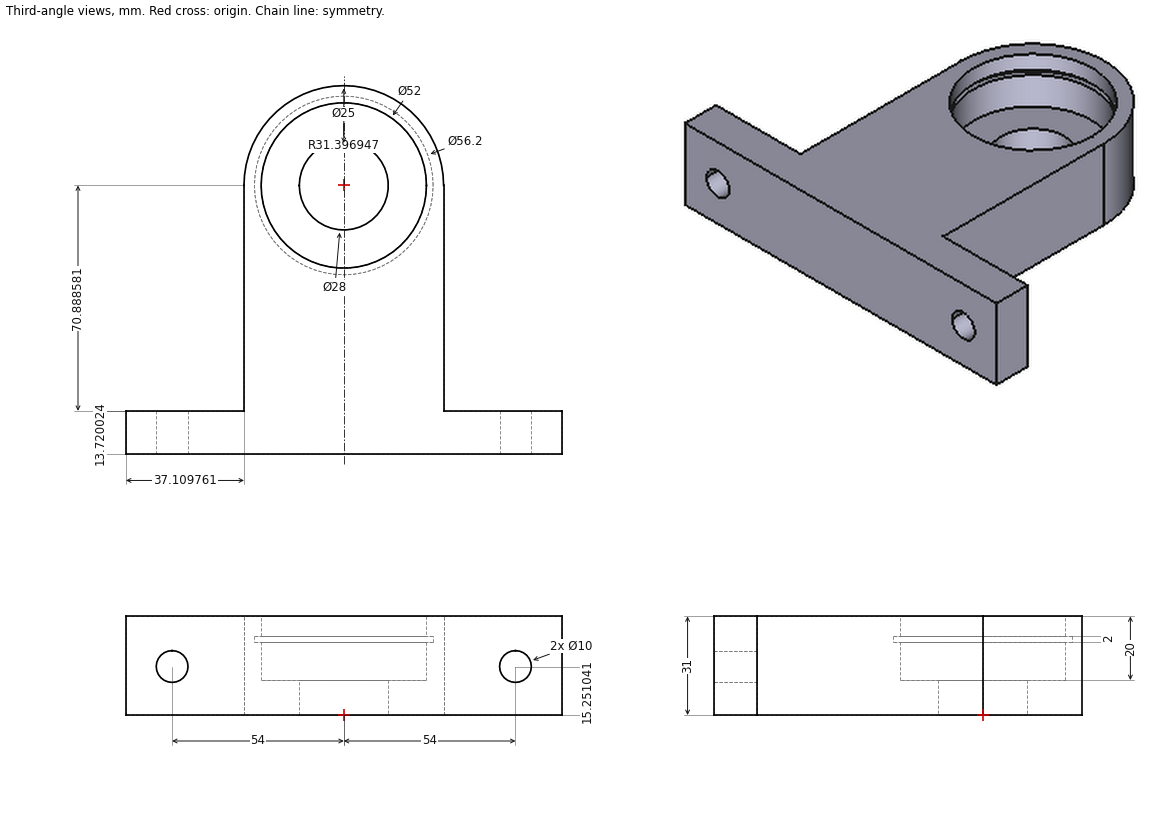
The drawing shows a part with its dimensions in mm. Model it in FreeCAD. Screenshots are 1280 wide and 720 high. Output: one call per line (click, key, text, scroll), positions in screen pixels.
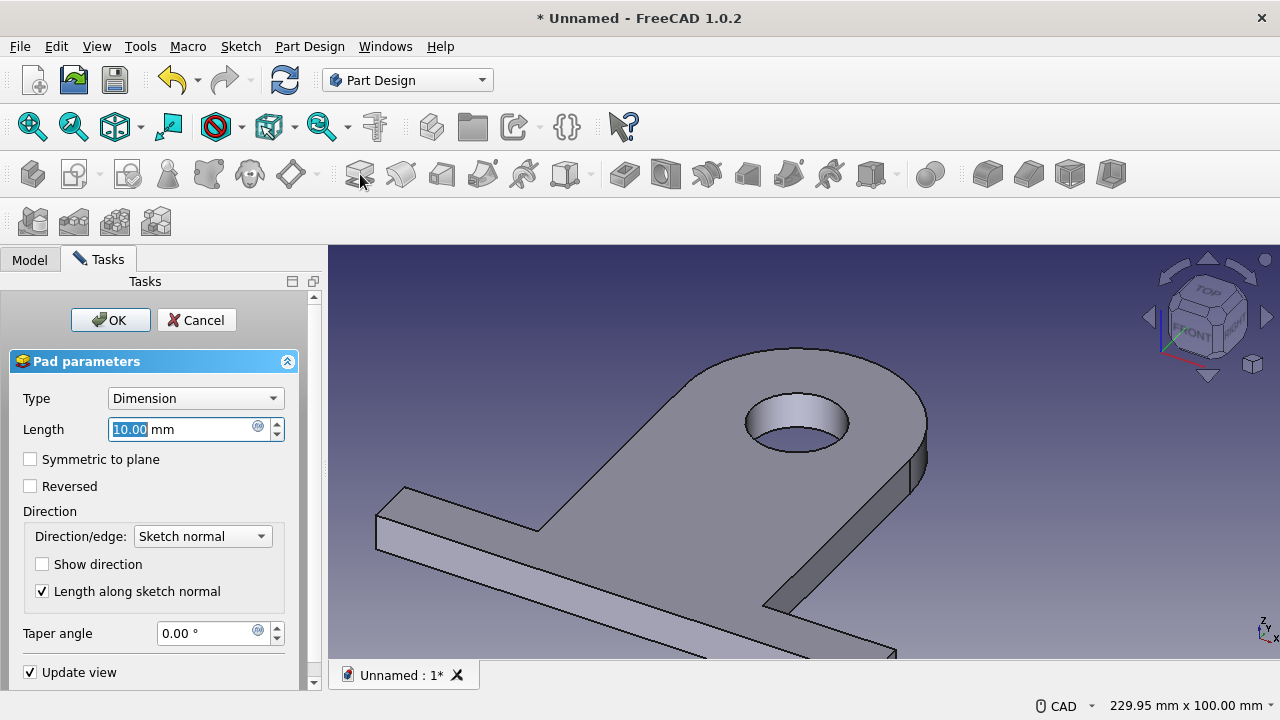
text(31)
key(Tab)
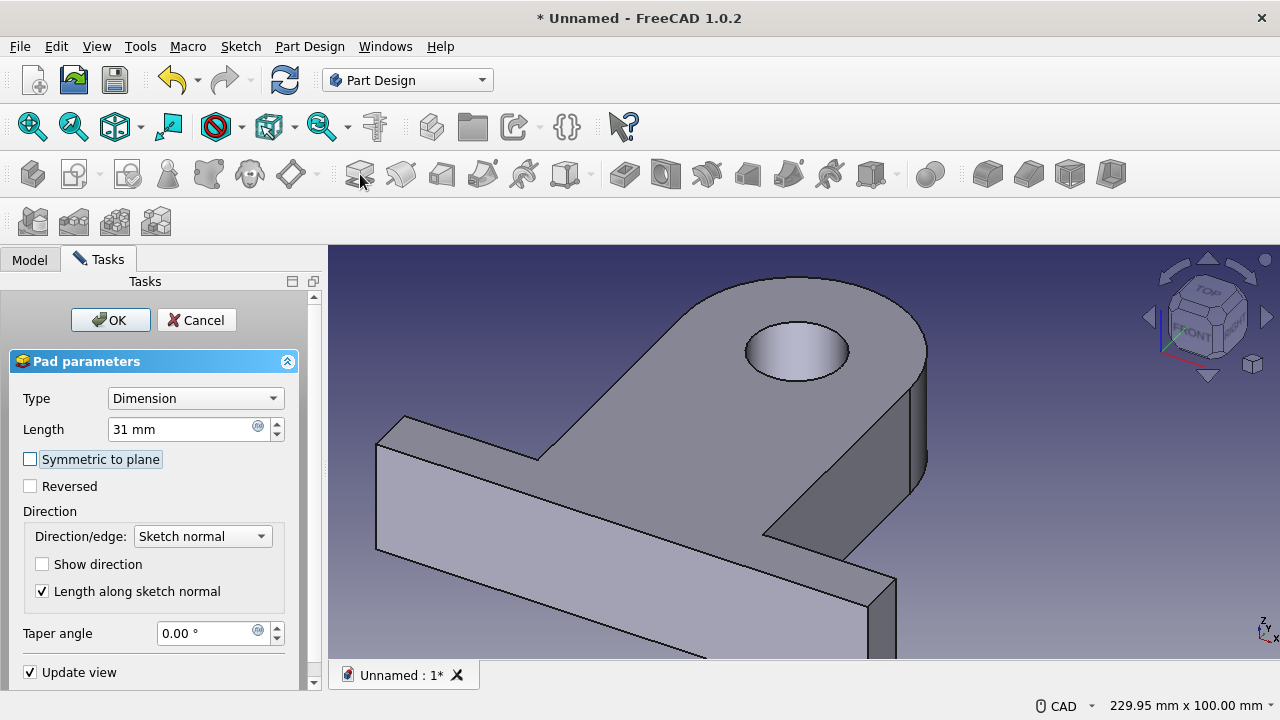
click(111, 320)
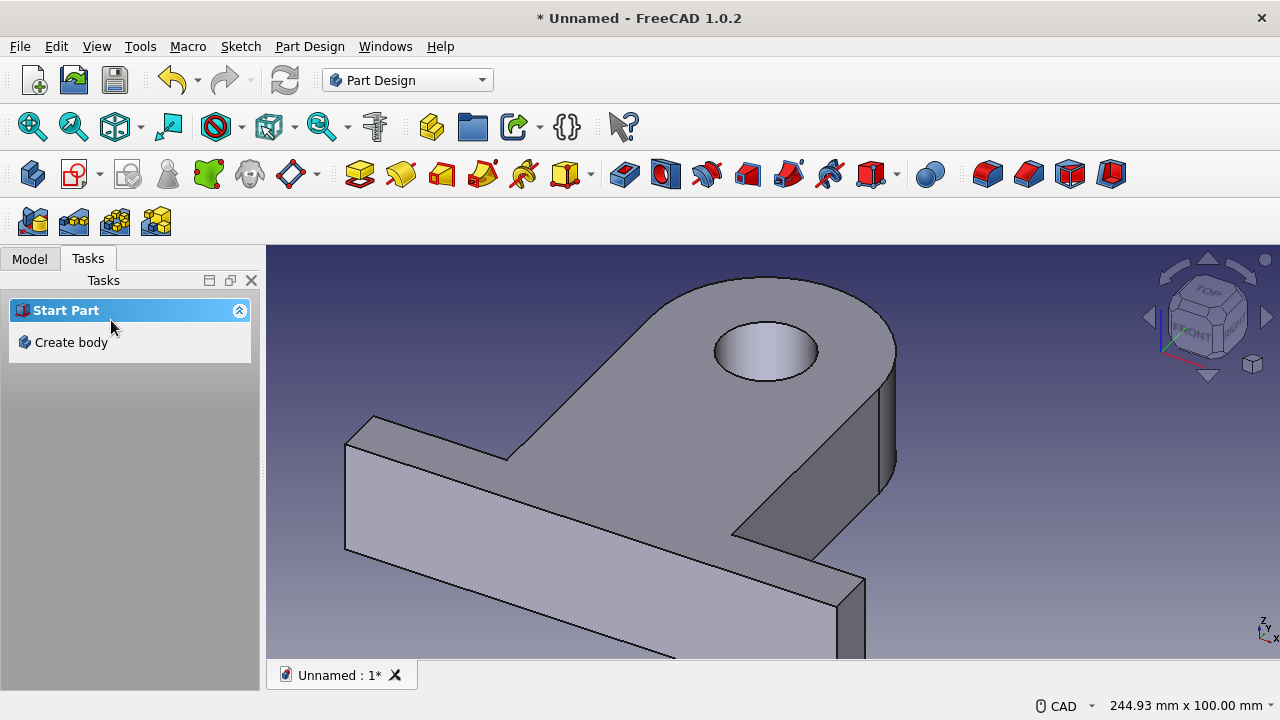
click(33, 128)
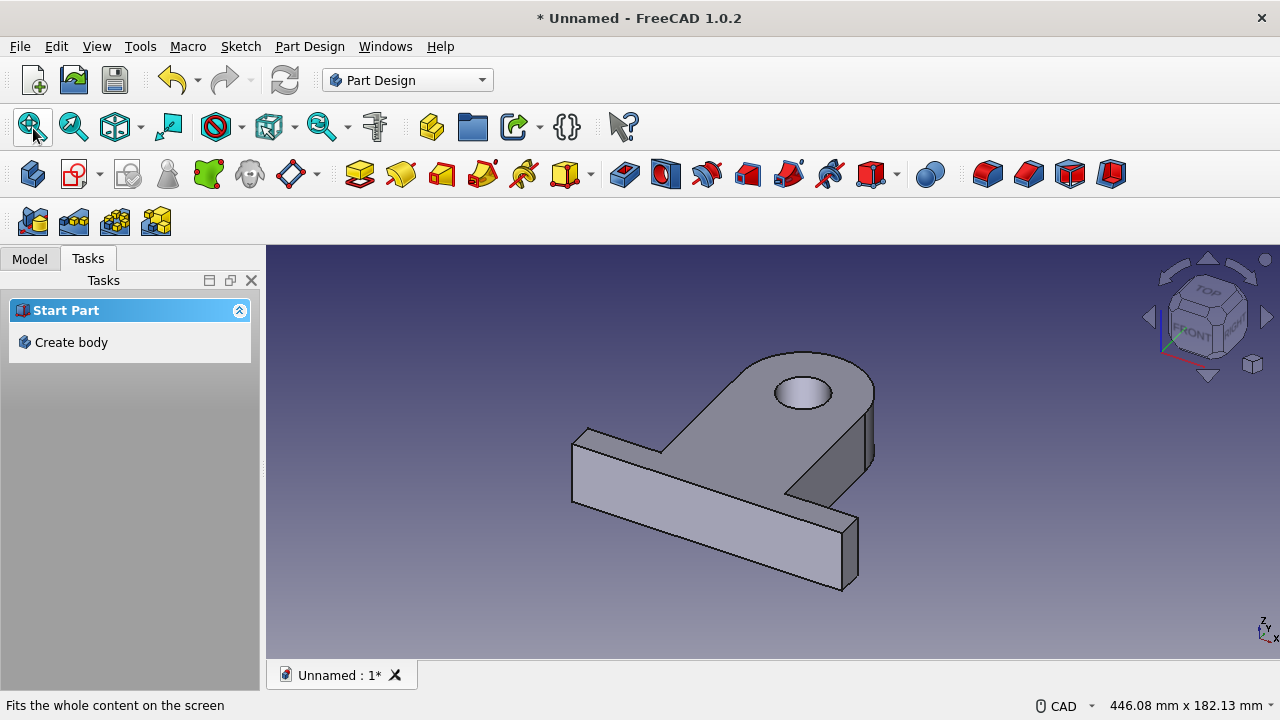
key(4)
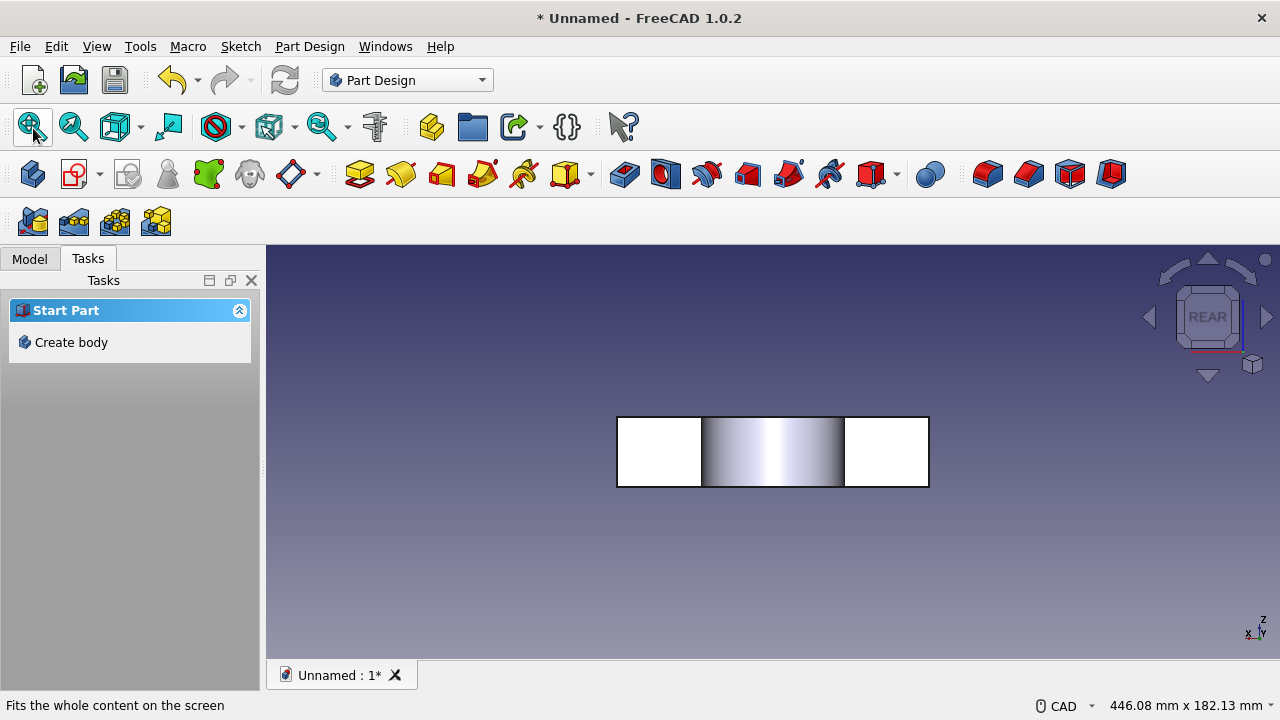
click(33, 128)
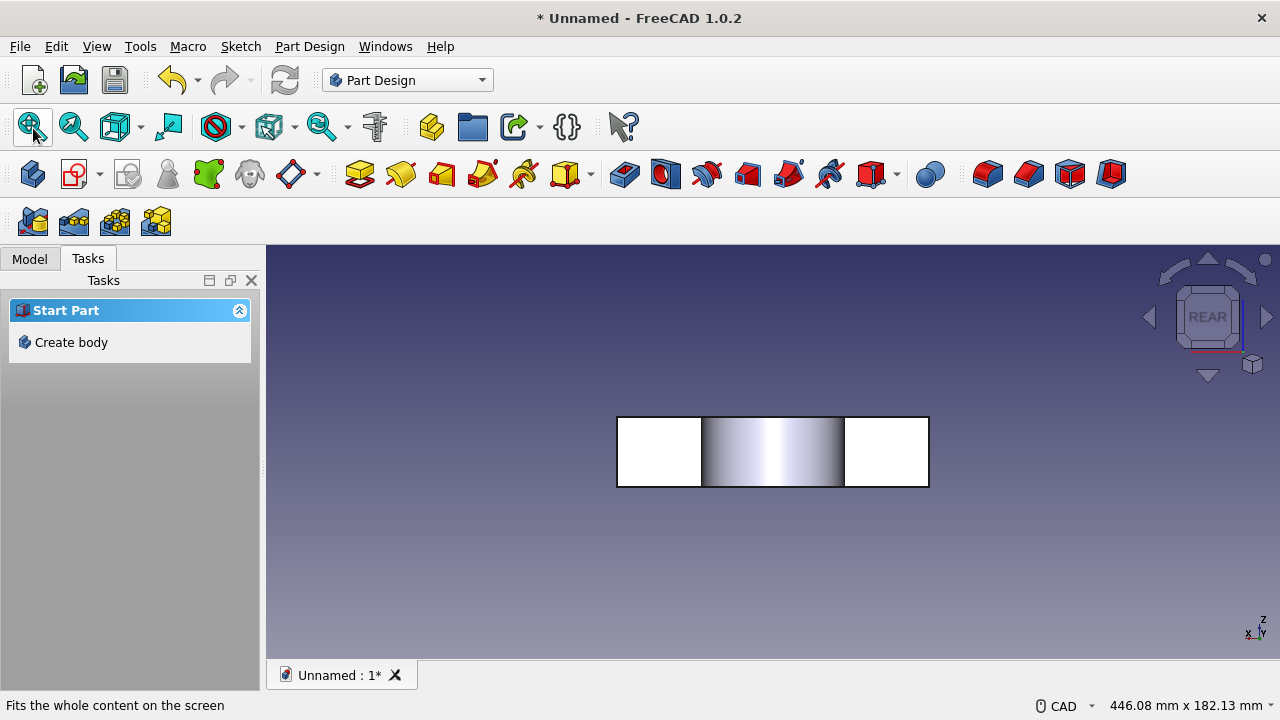
click(659, 451)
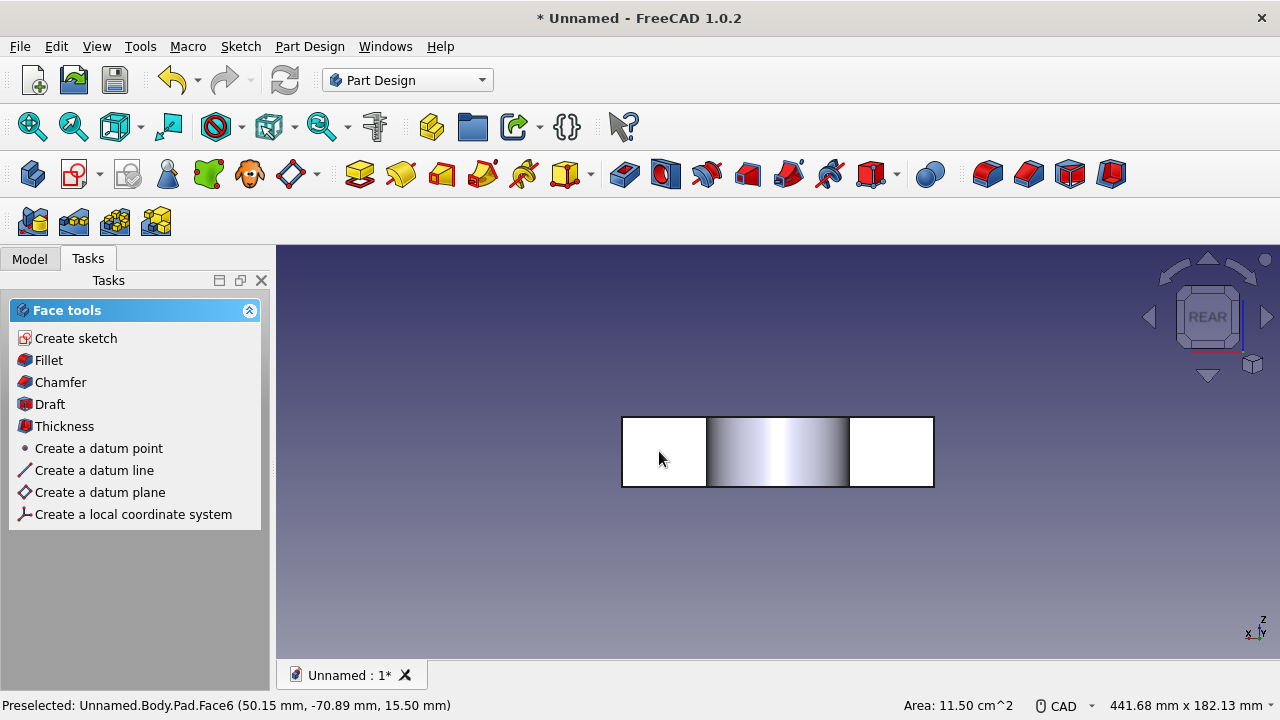
click(74, 174)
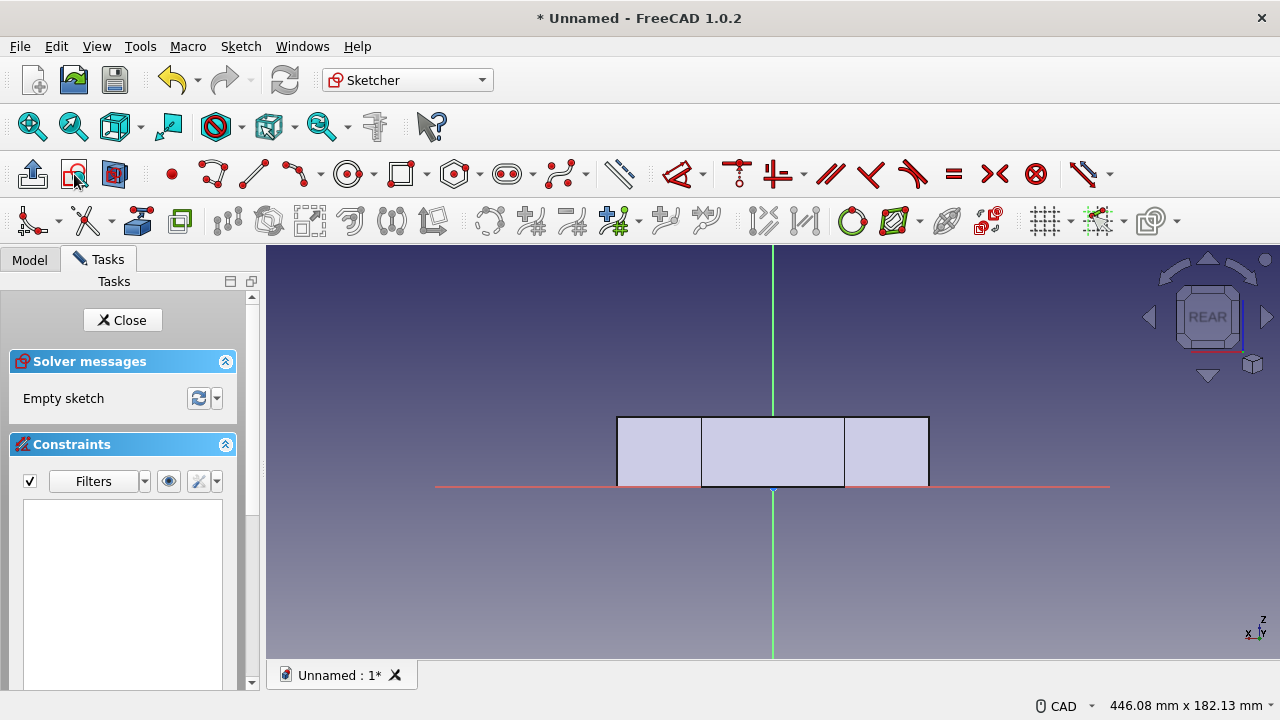
scroll(829, 474, up, 4)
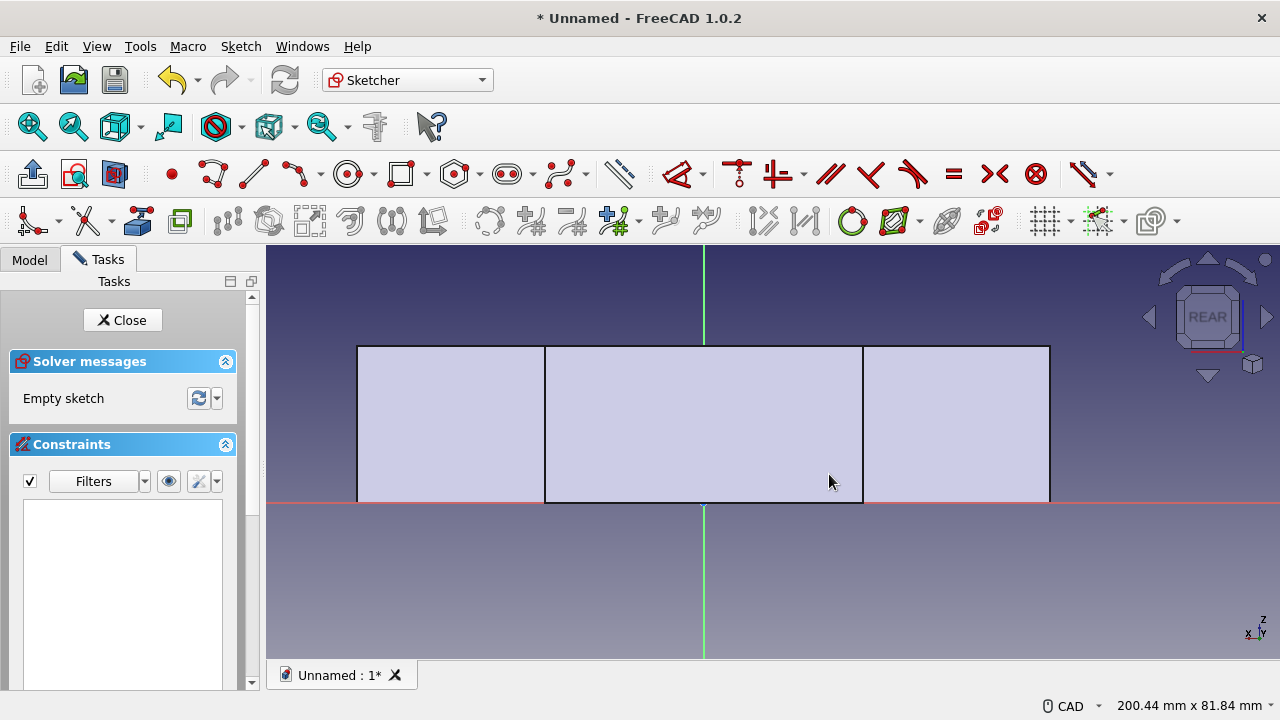
click(348, 174)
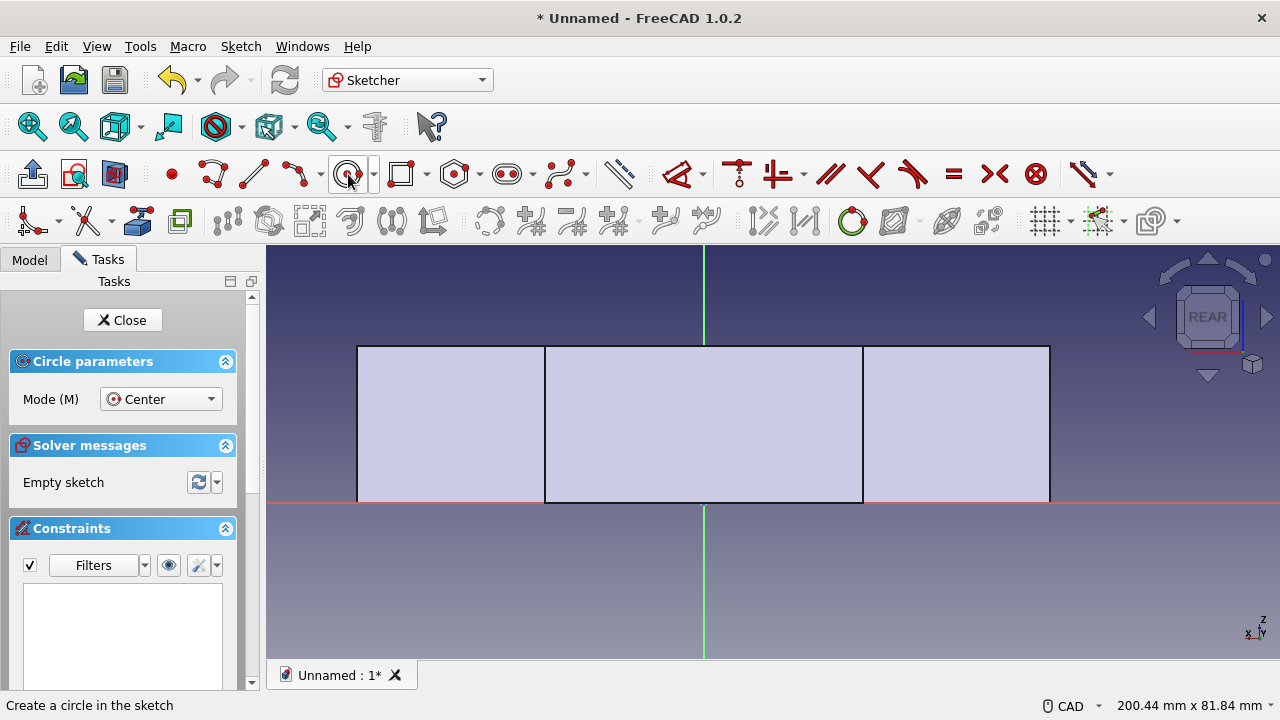
click(431, 426)
click(448, 408)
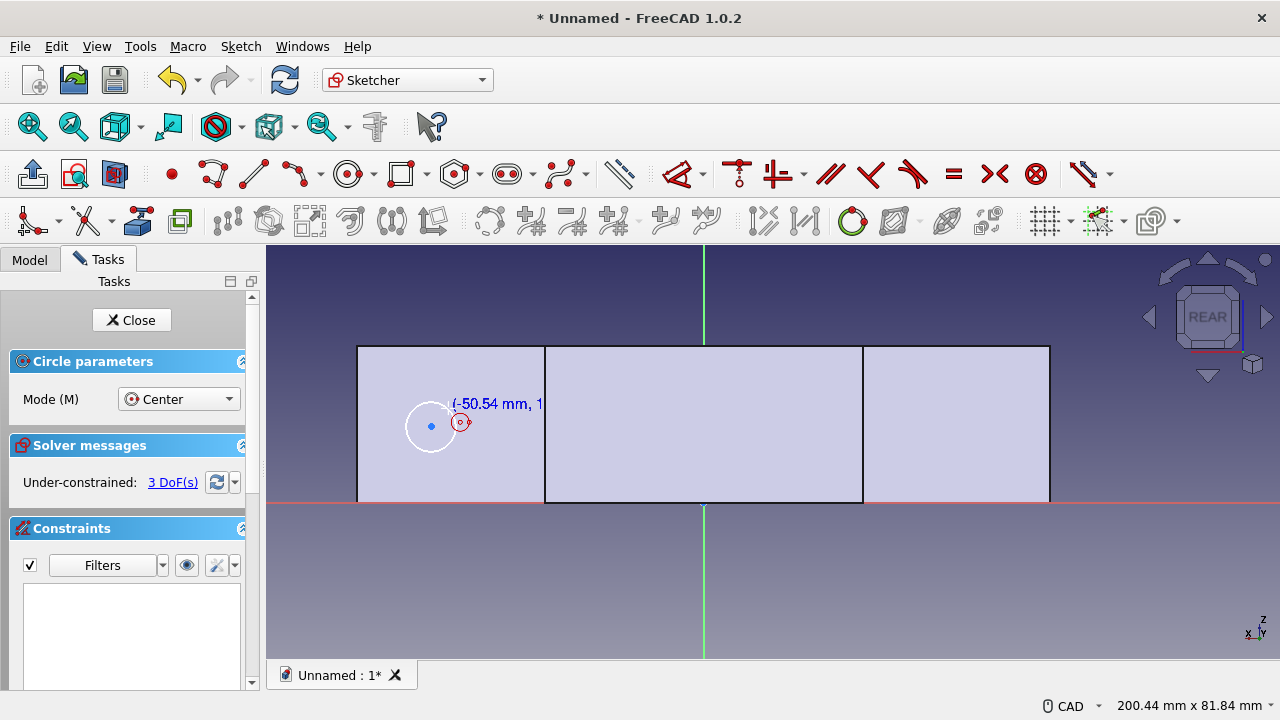
click(977, 426)
click(995, 408)
key(Escape)